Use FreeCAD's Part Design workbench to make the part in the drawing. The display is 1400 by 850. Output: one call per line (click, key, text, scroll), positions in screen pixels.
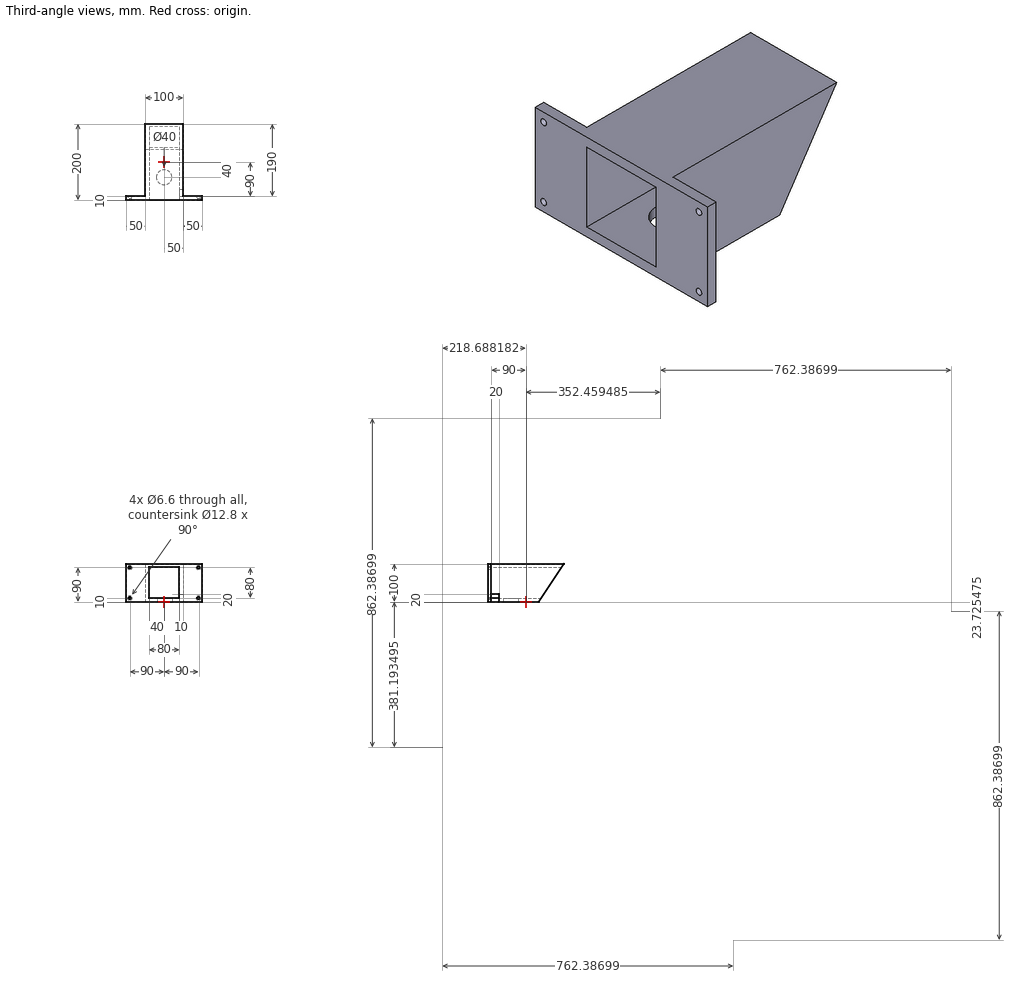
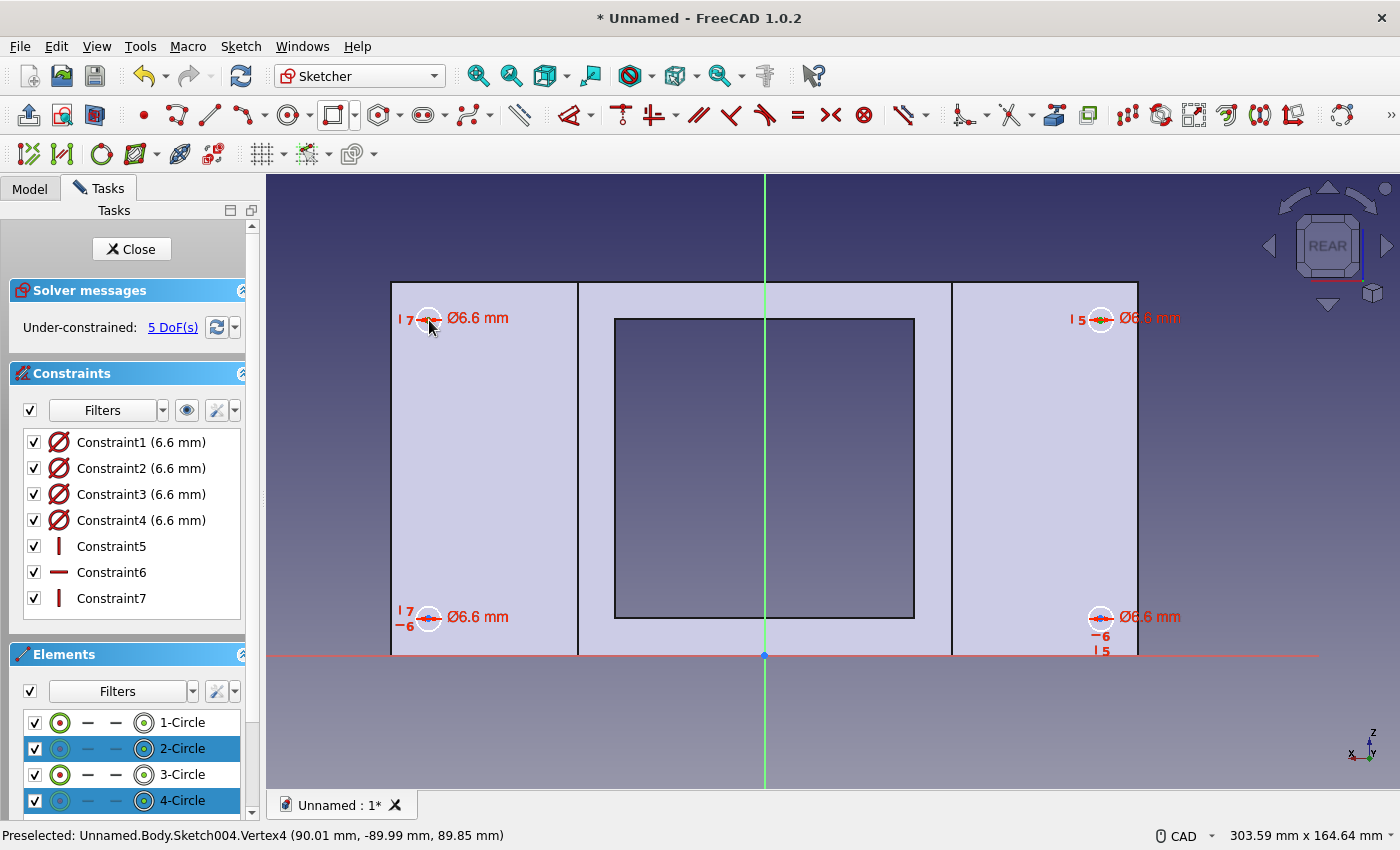
click(676, 116)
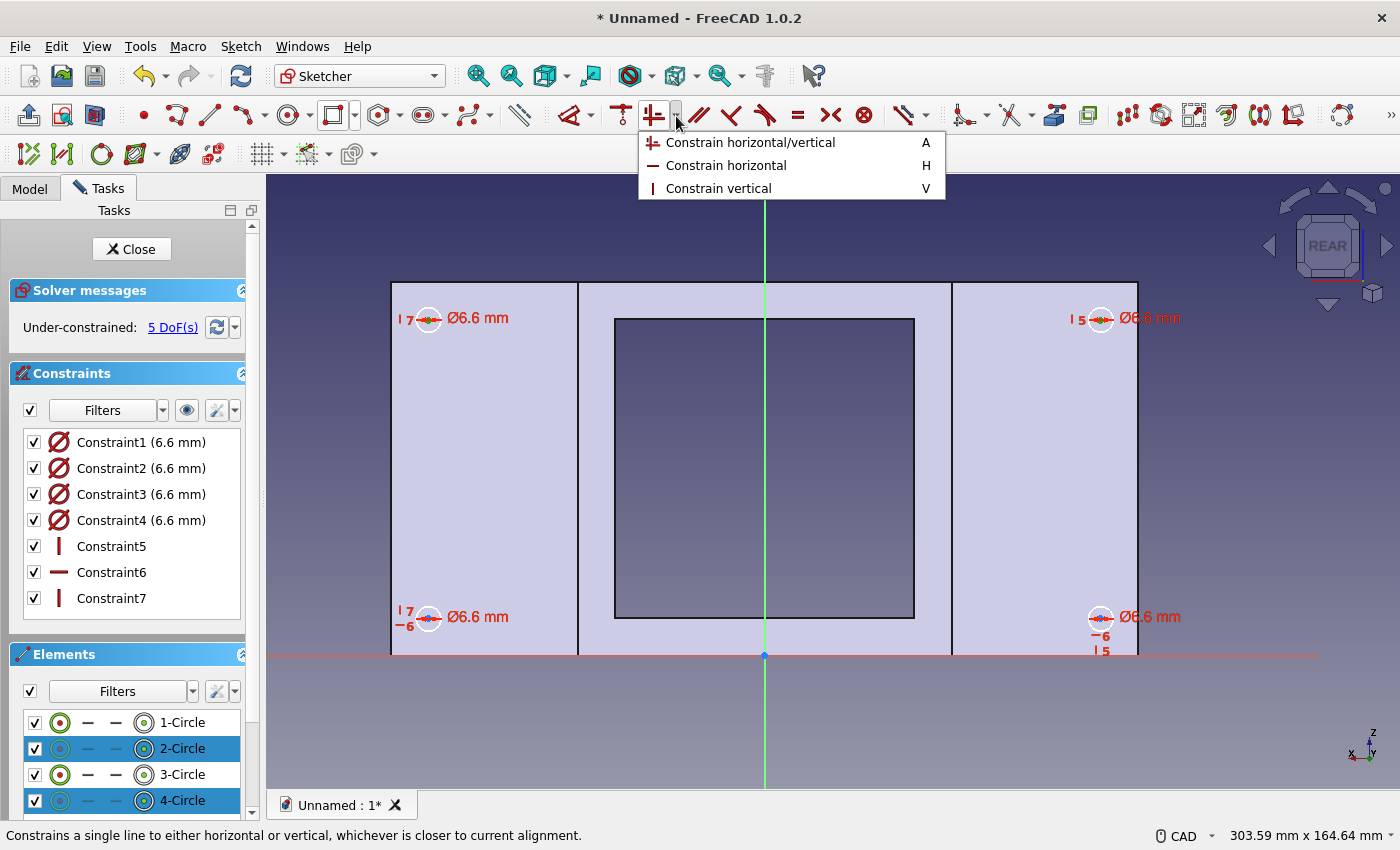
click(792, 166)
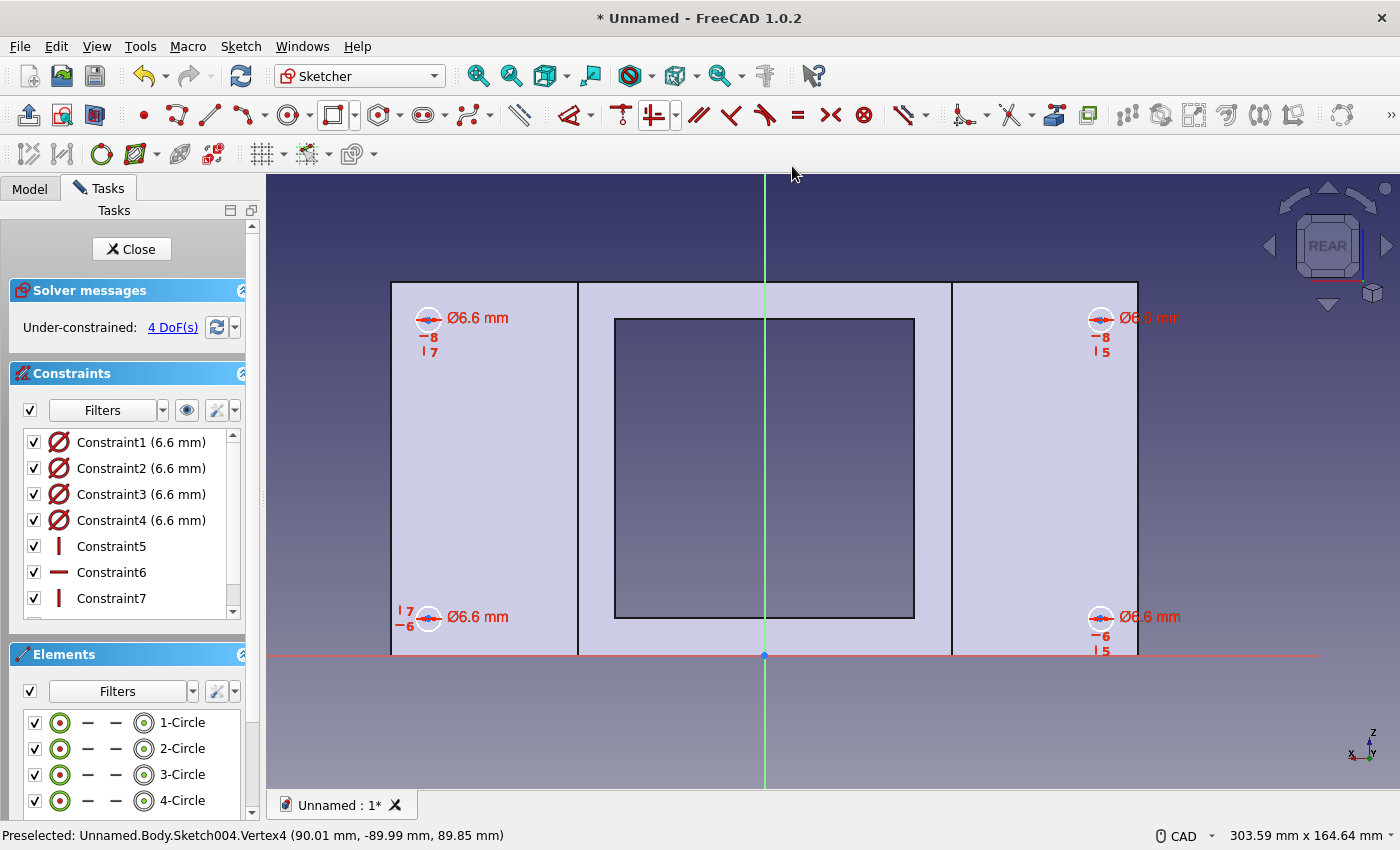
key(d)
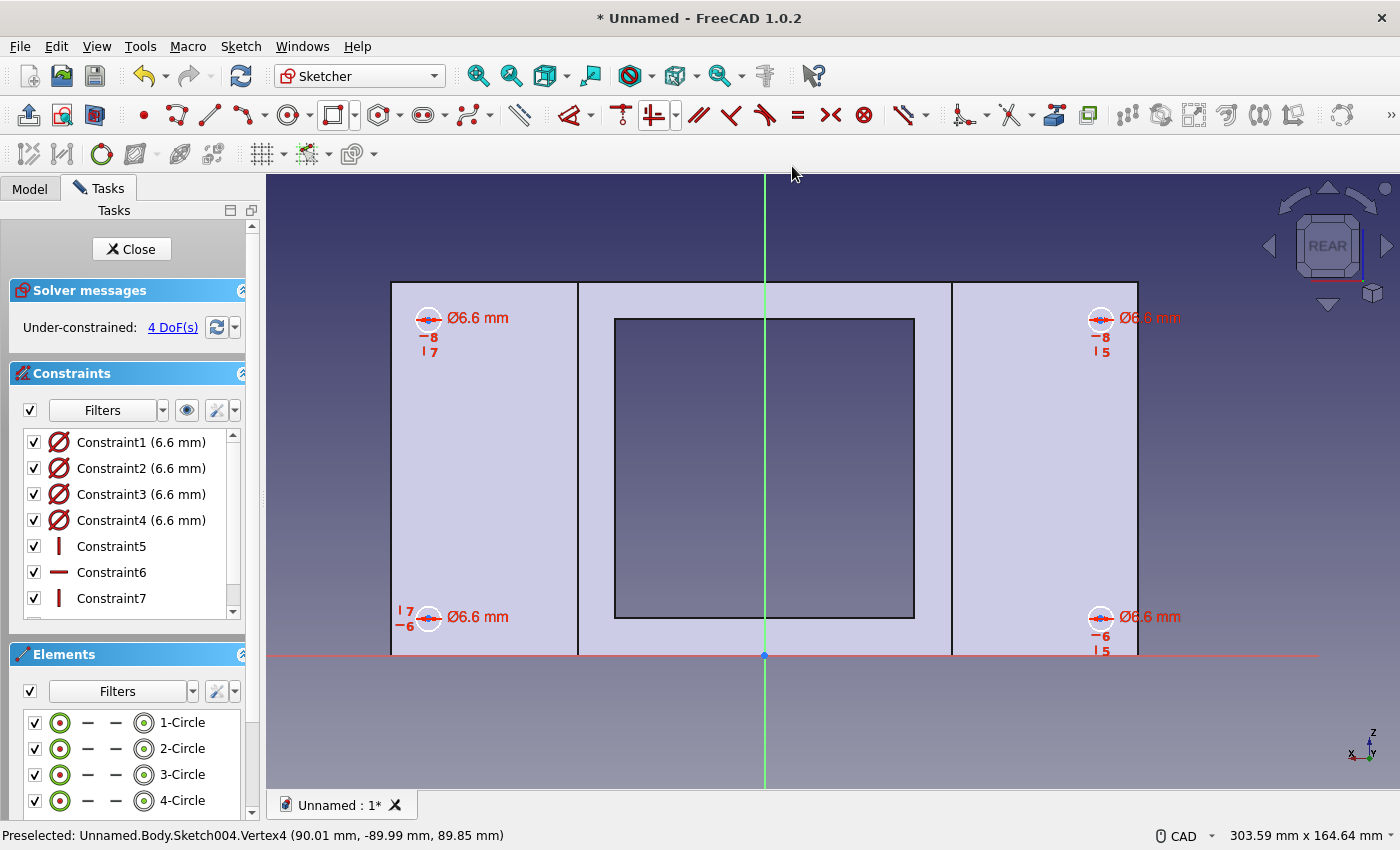
click(1101, 619)
click(933, 690)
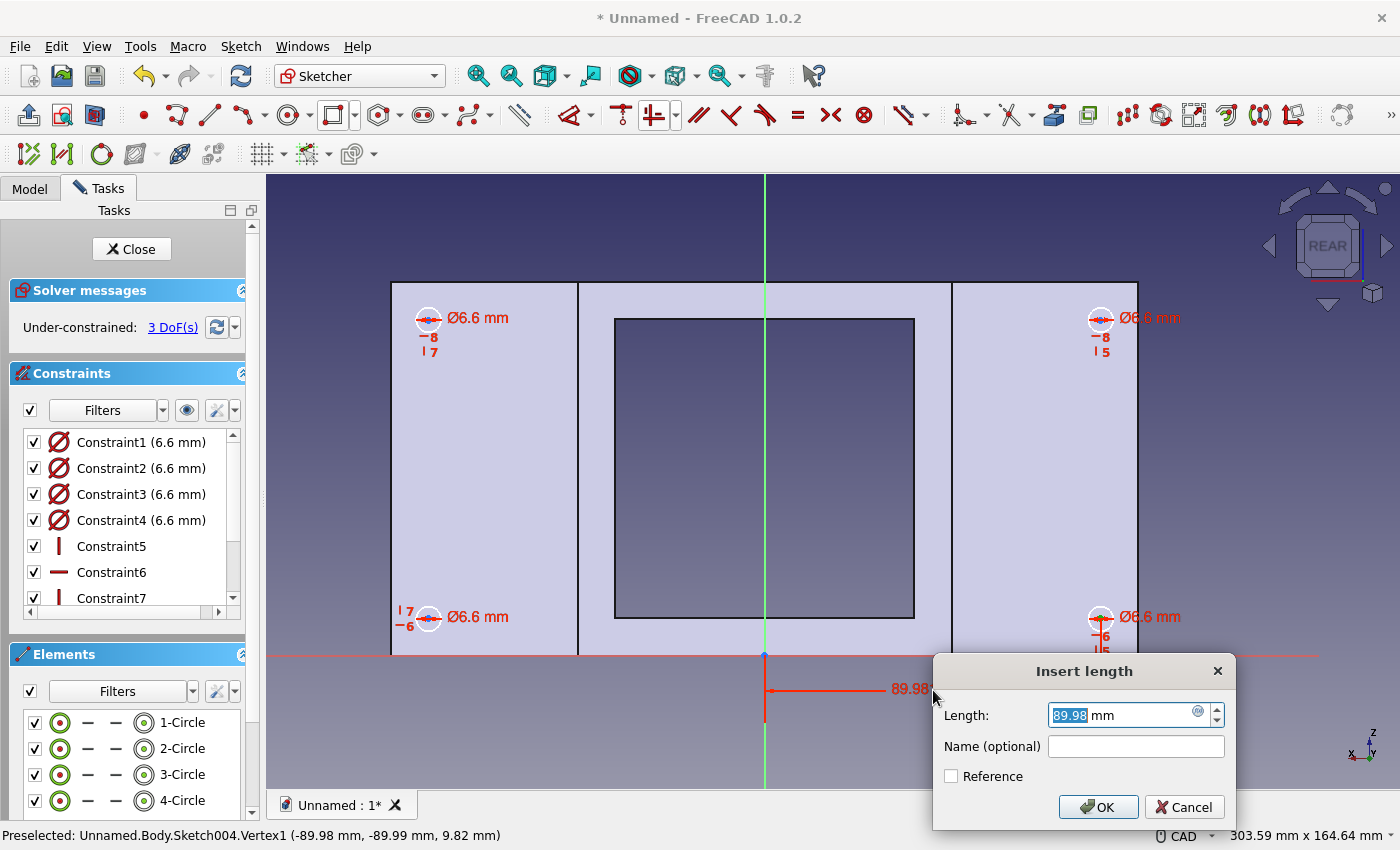
text(90)
key(Return)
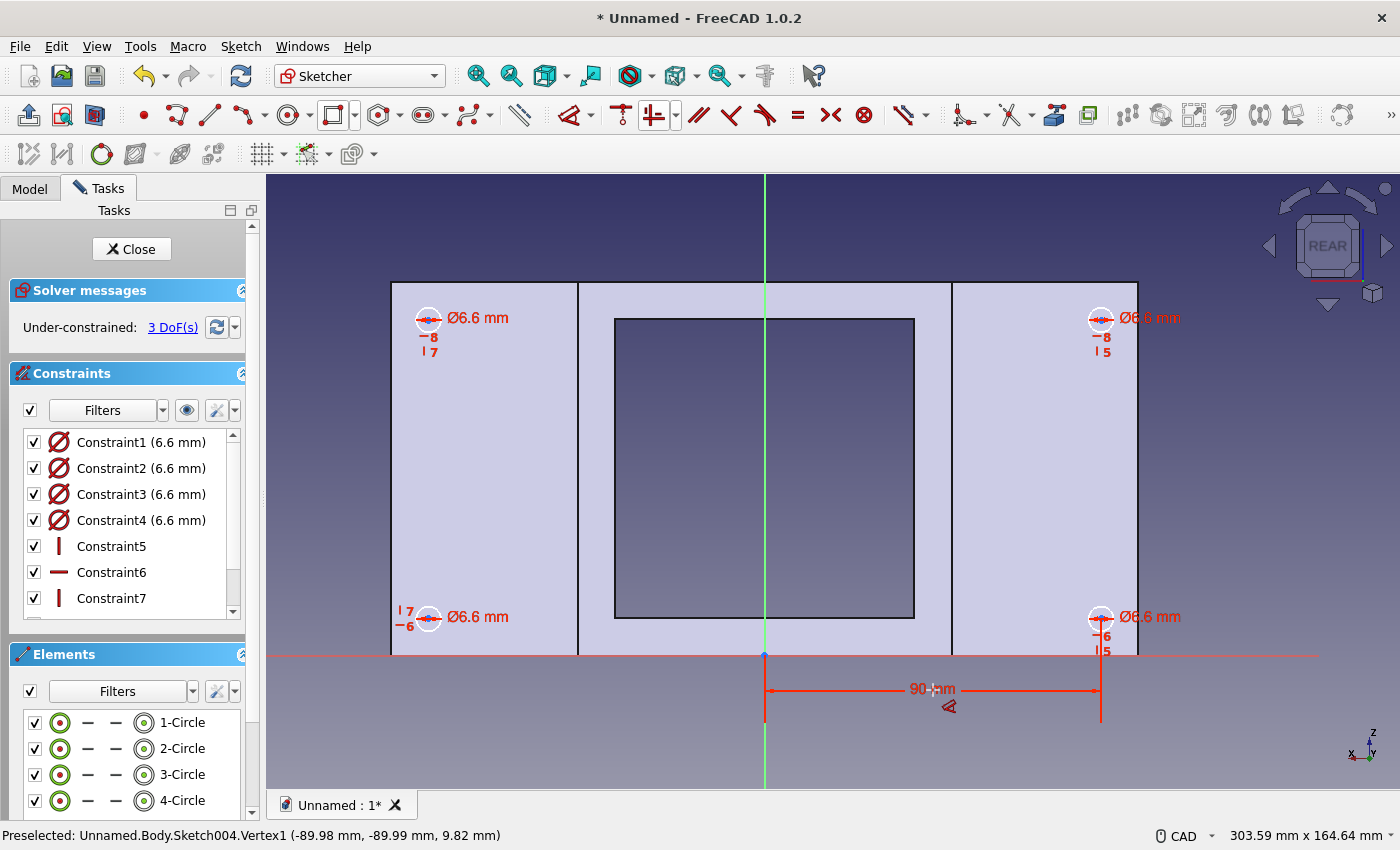
click(1101, 619)
click(1135, 637)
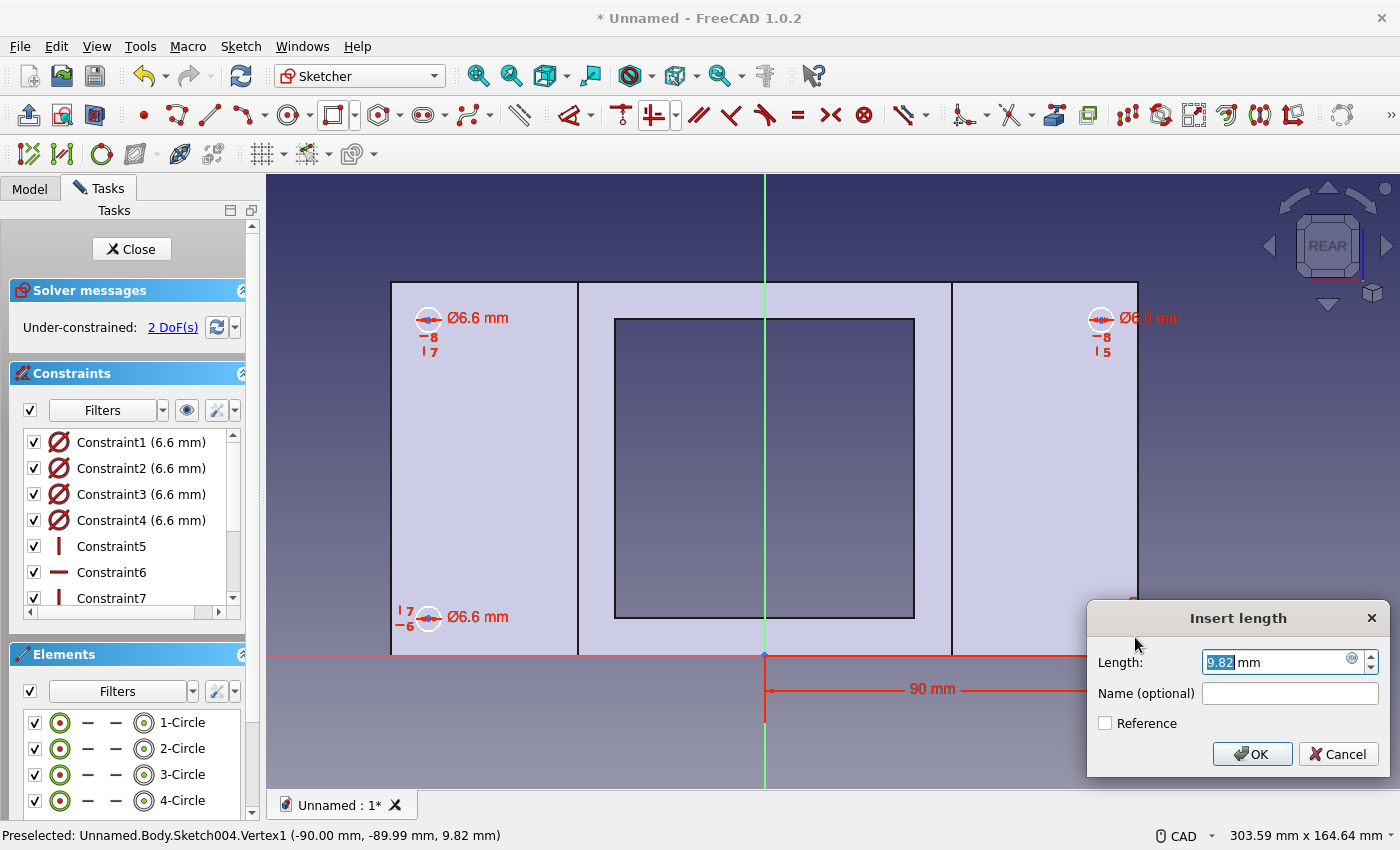
text(10)
key(Return)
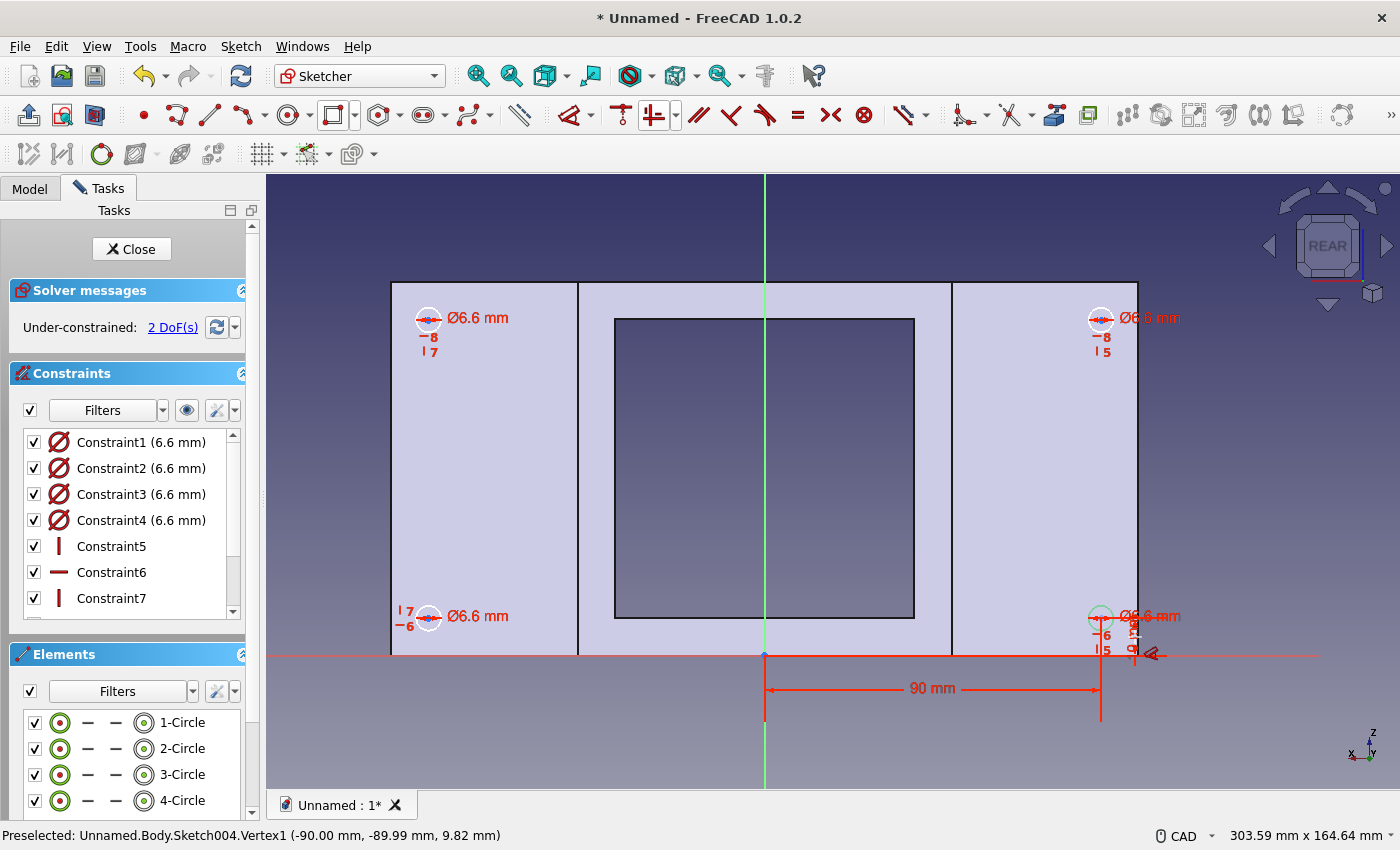
click(1101, 320)
click(1135, 488)